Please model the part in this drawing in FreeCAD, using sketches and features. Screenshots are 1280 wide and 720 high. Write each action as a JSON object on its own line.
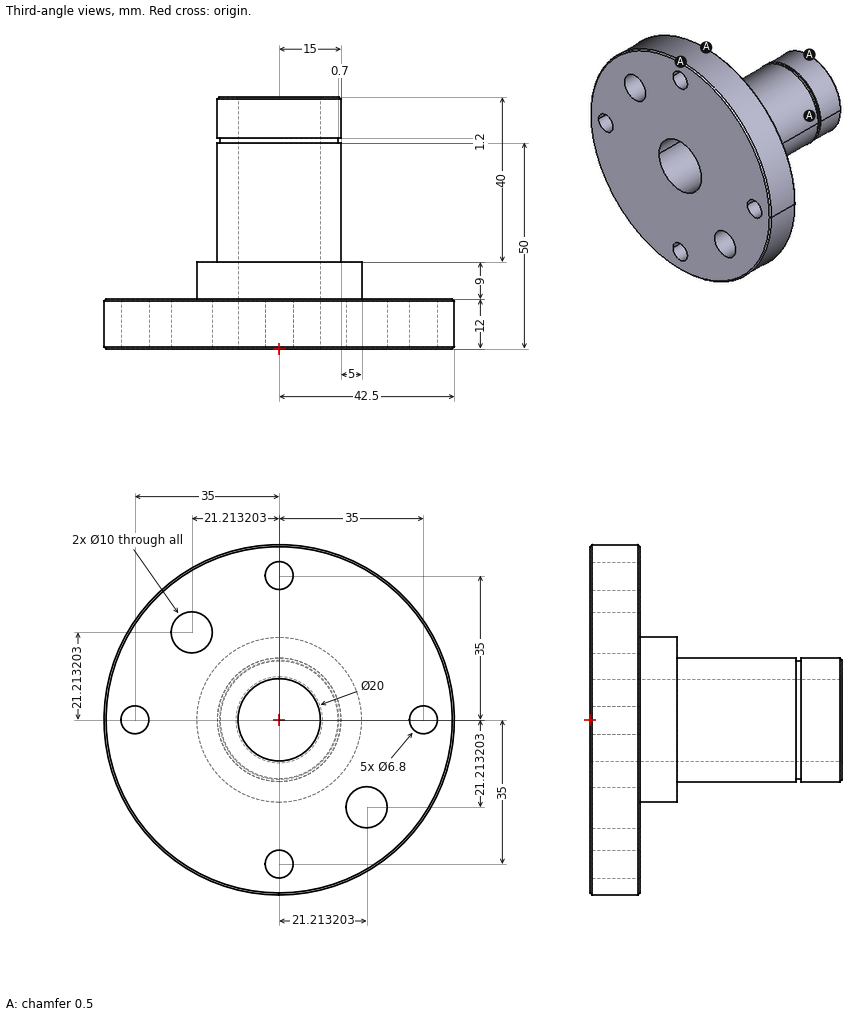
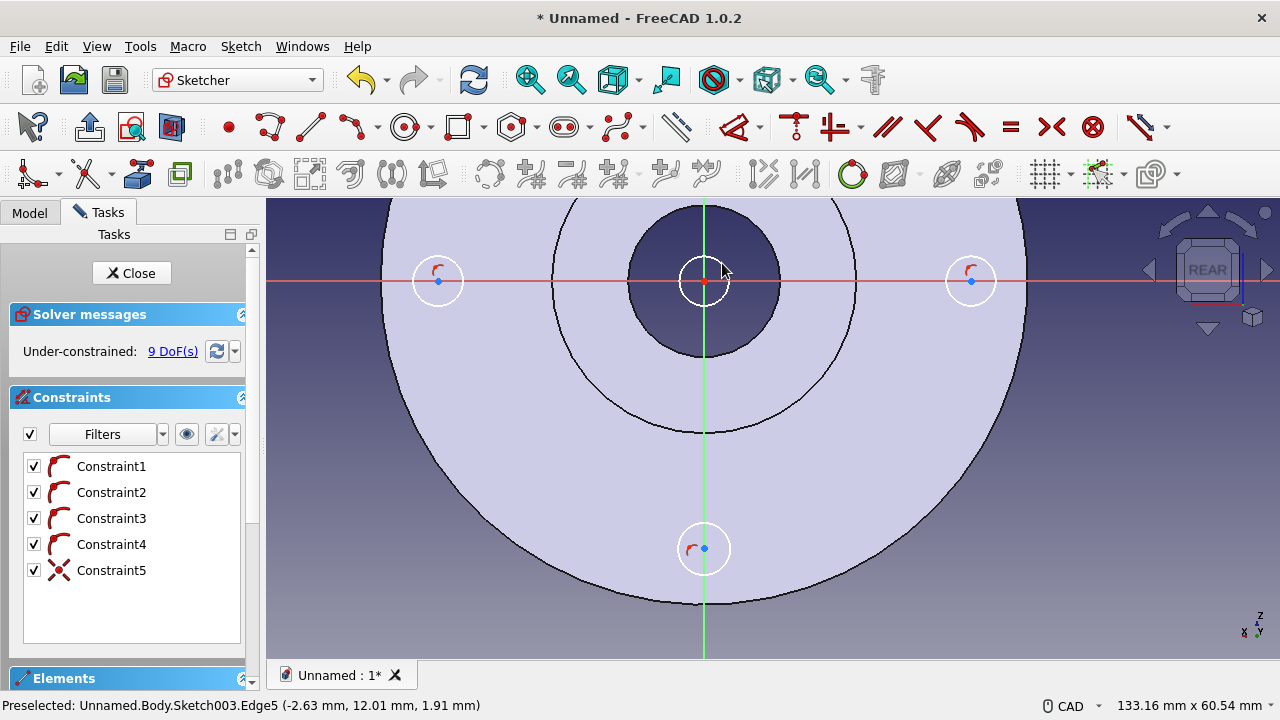
{"action": "left_click", "coordinate": [456, 263]}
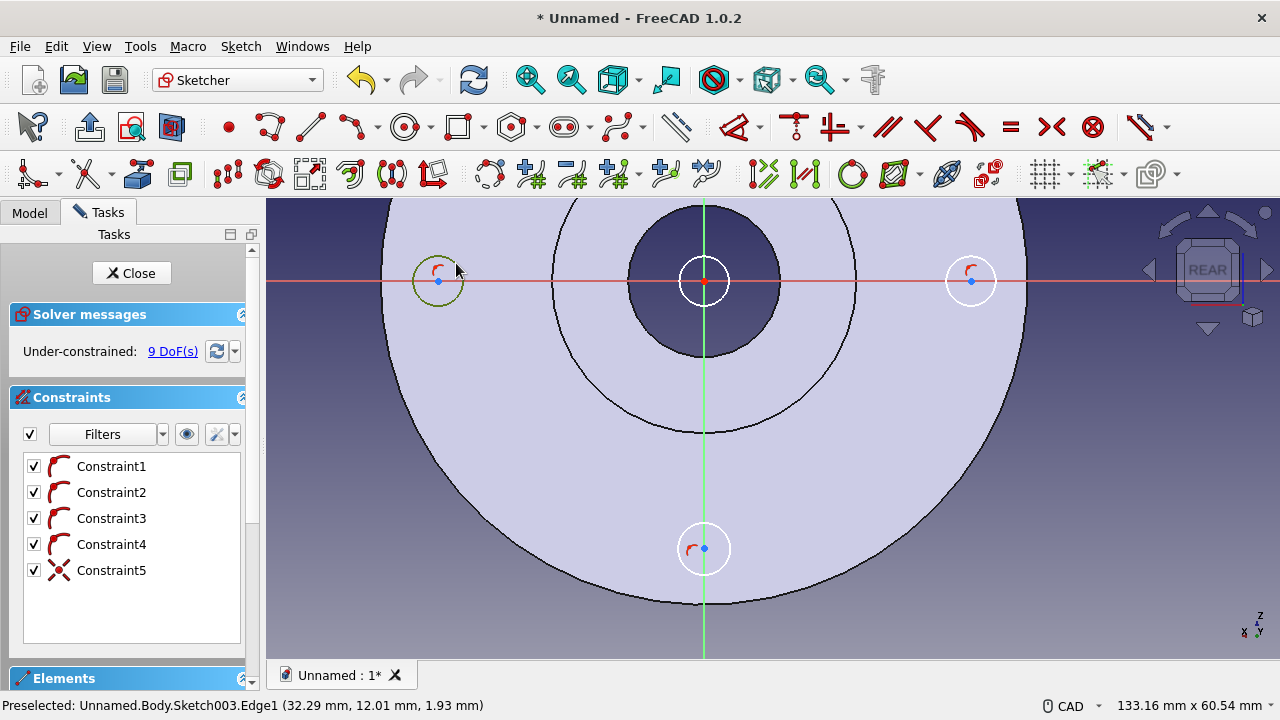
{"action": "scroll", "coordinate": [705, 549], "scroll_direction": "down", "scroll_amount": 4}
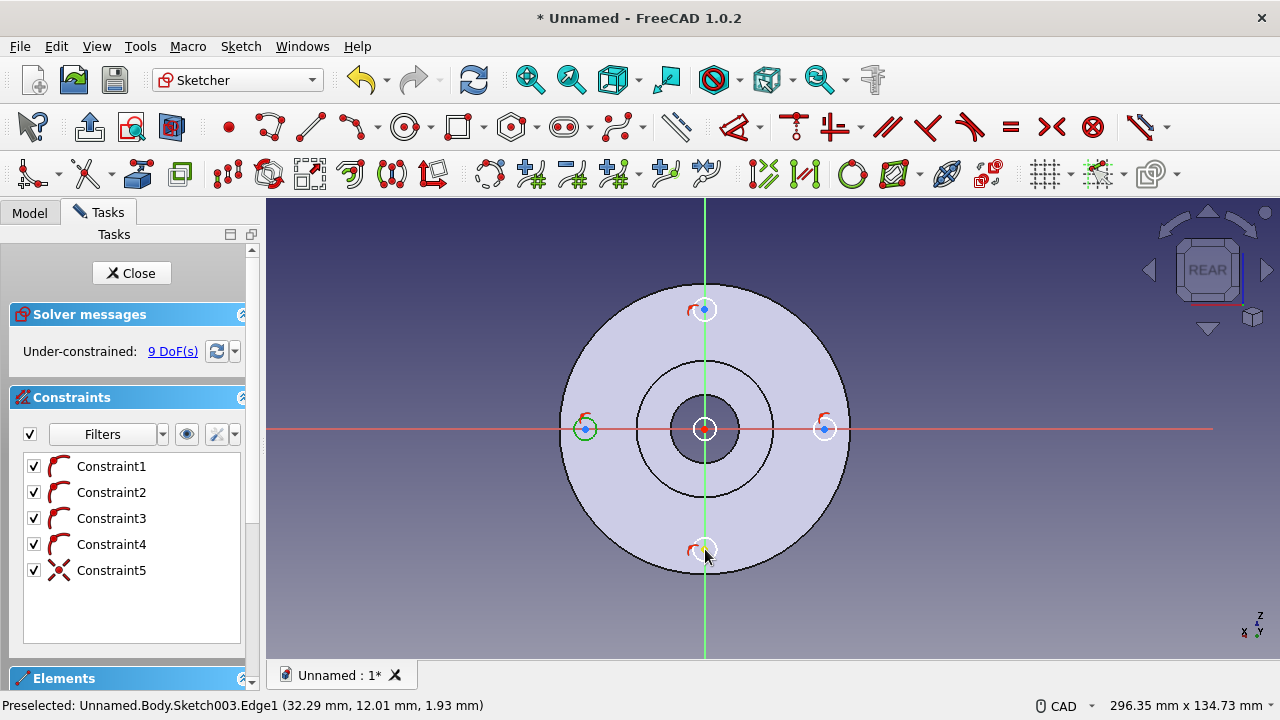
{"action": "scroll", "coordinate": [713, 302], "scroll_direction": "up", "scroll_amount": 3}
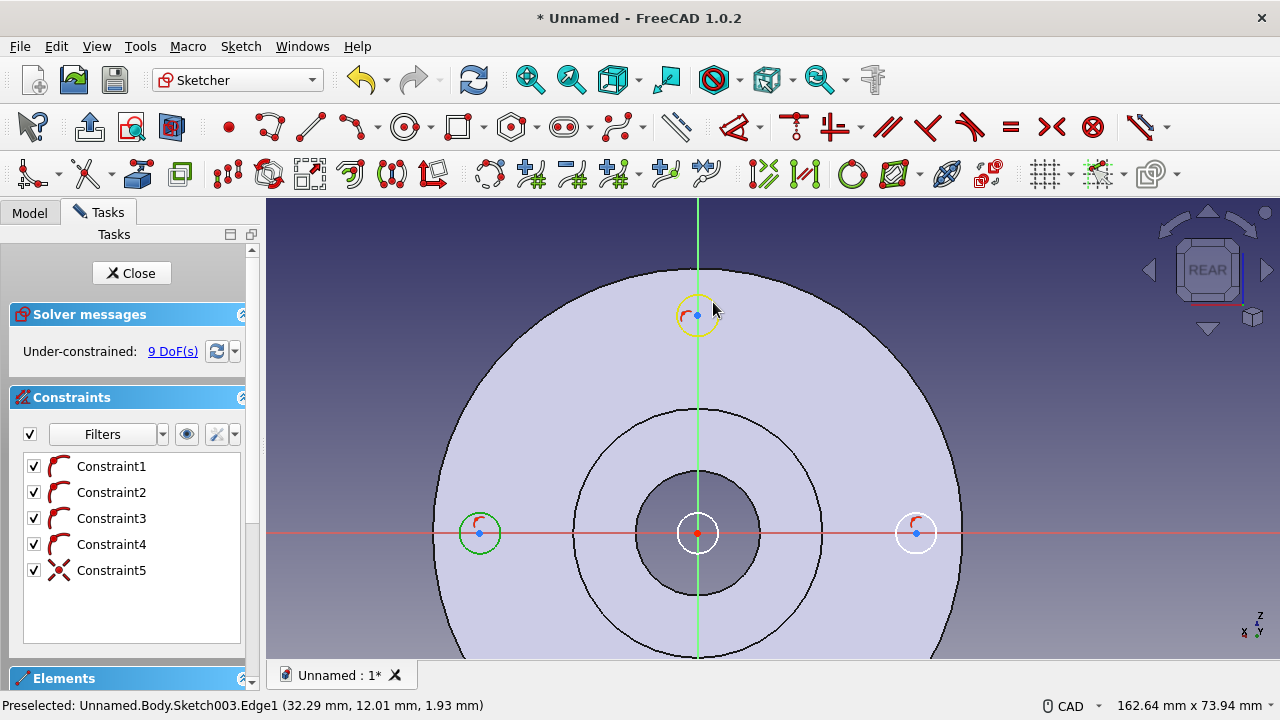
{"action": "left_click", "coordinate": [712, 301]}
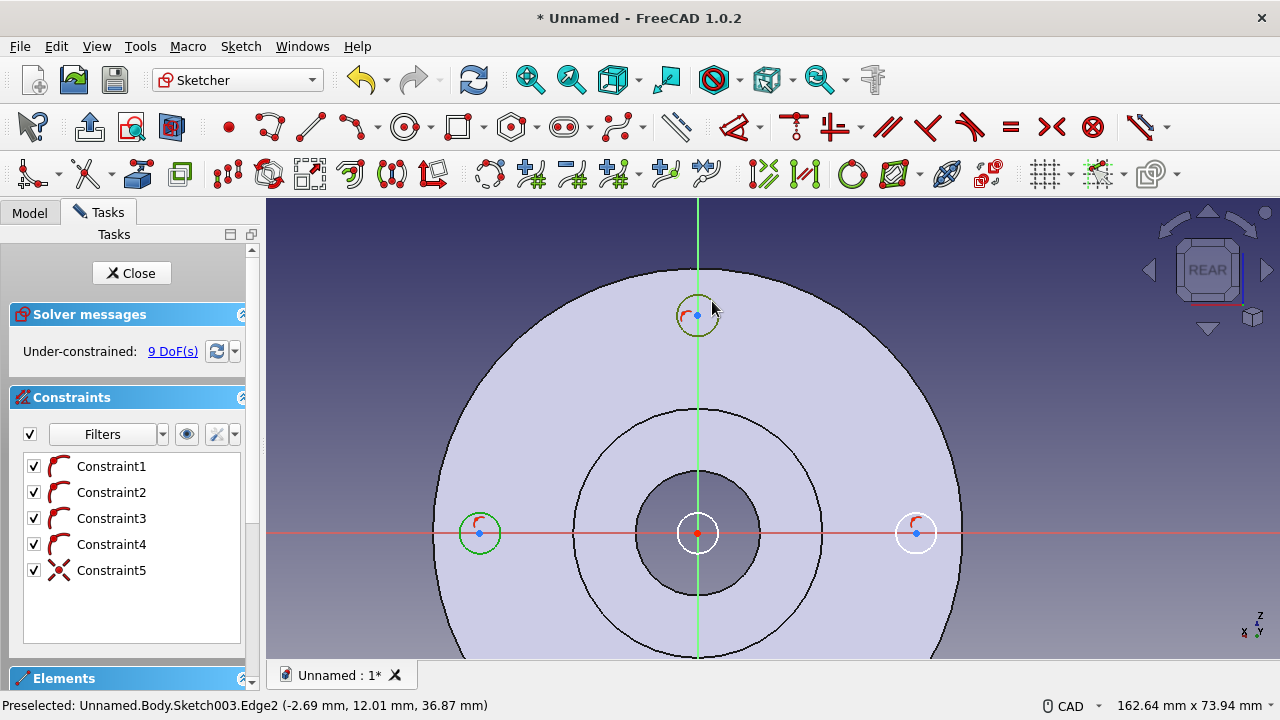
{"action": "left_click", "coordinate": [931, 519]}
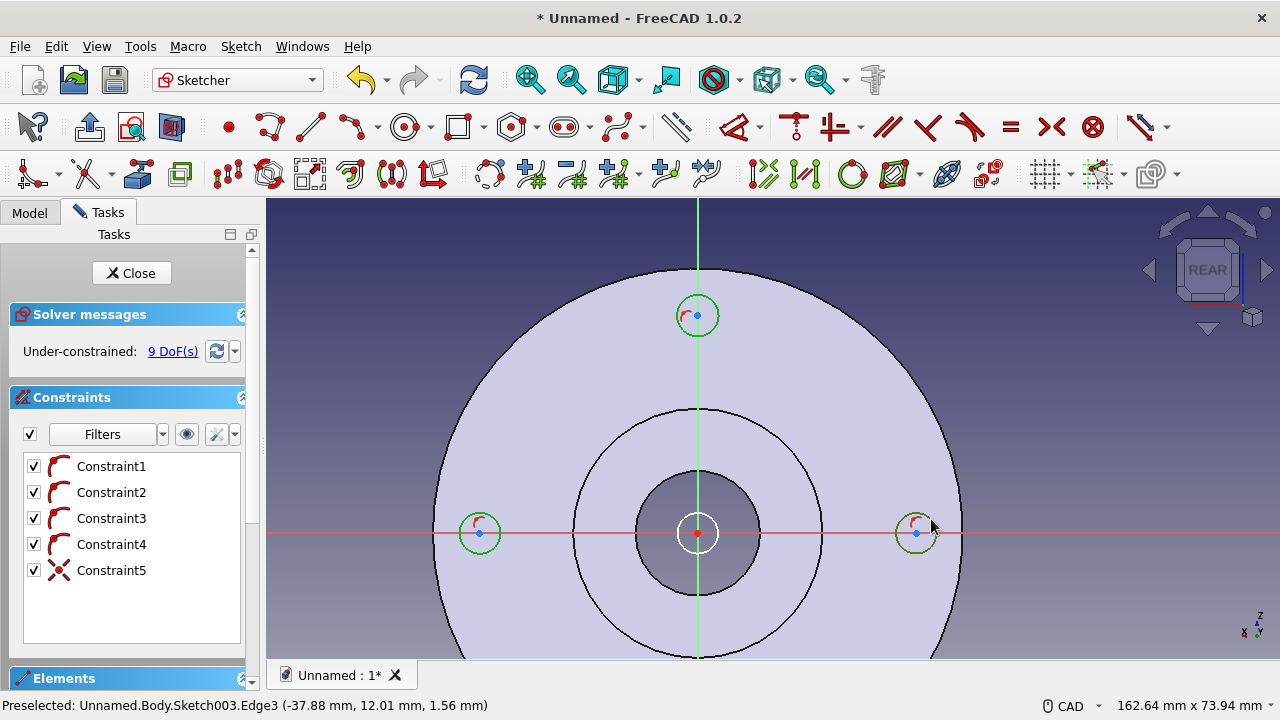
{"action": "scroll", "coordinate": [713, 301], "scroll_direction": "down", "scroll_amount": 3}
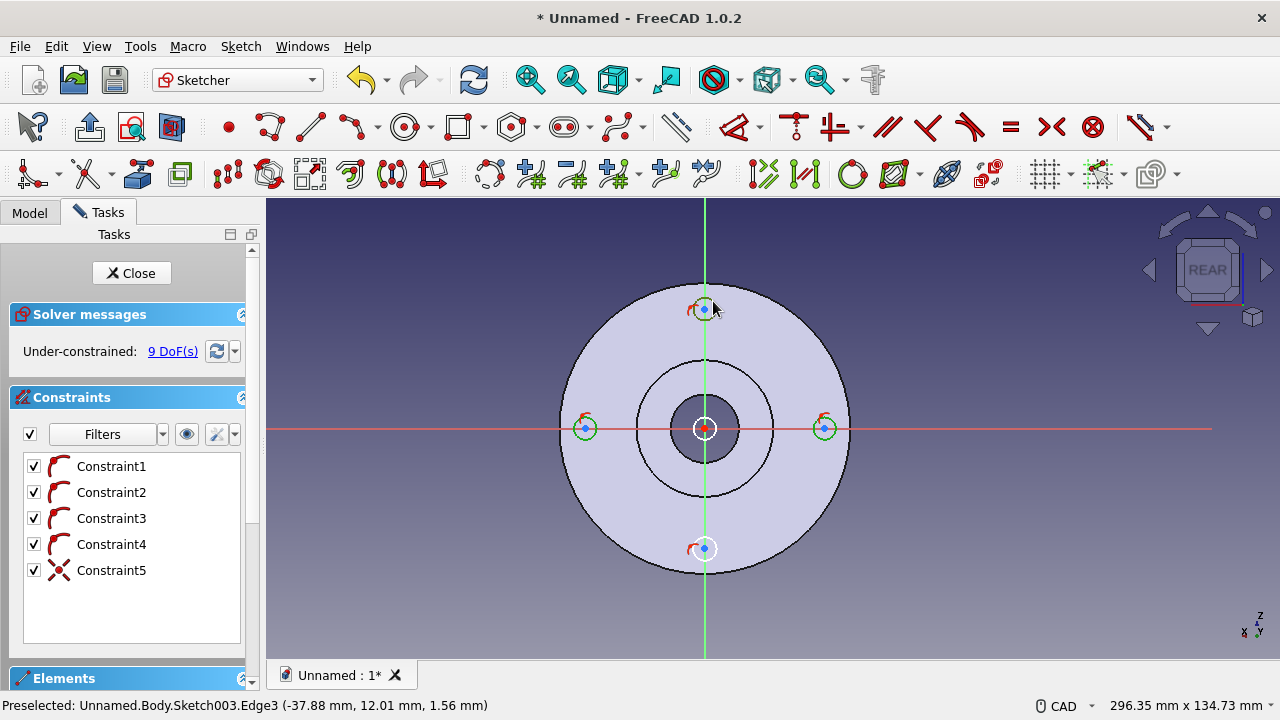
{"action": "scroll", "coordinate": [713, 541], "scroll_direction": "up", "scroll_amount": 3}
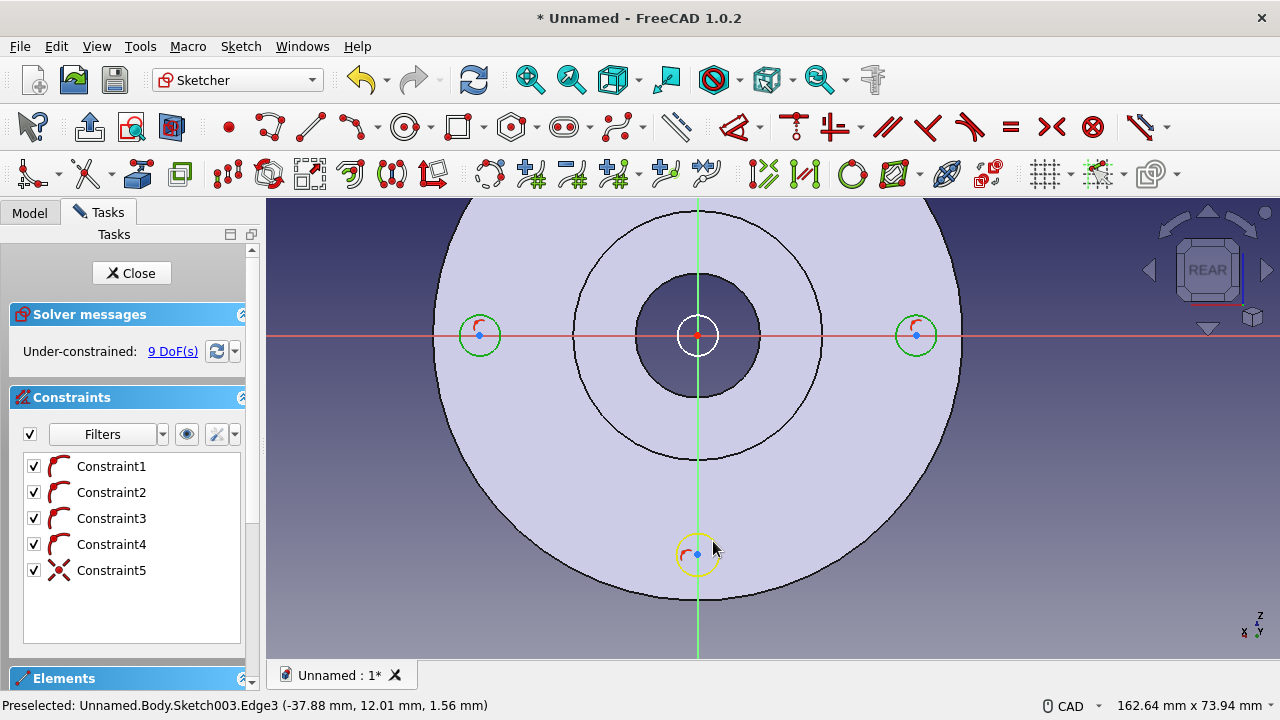
{"action": "left_click", "coordinate": [713, 540]}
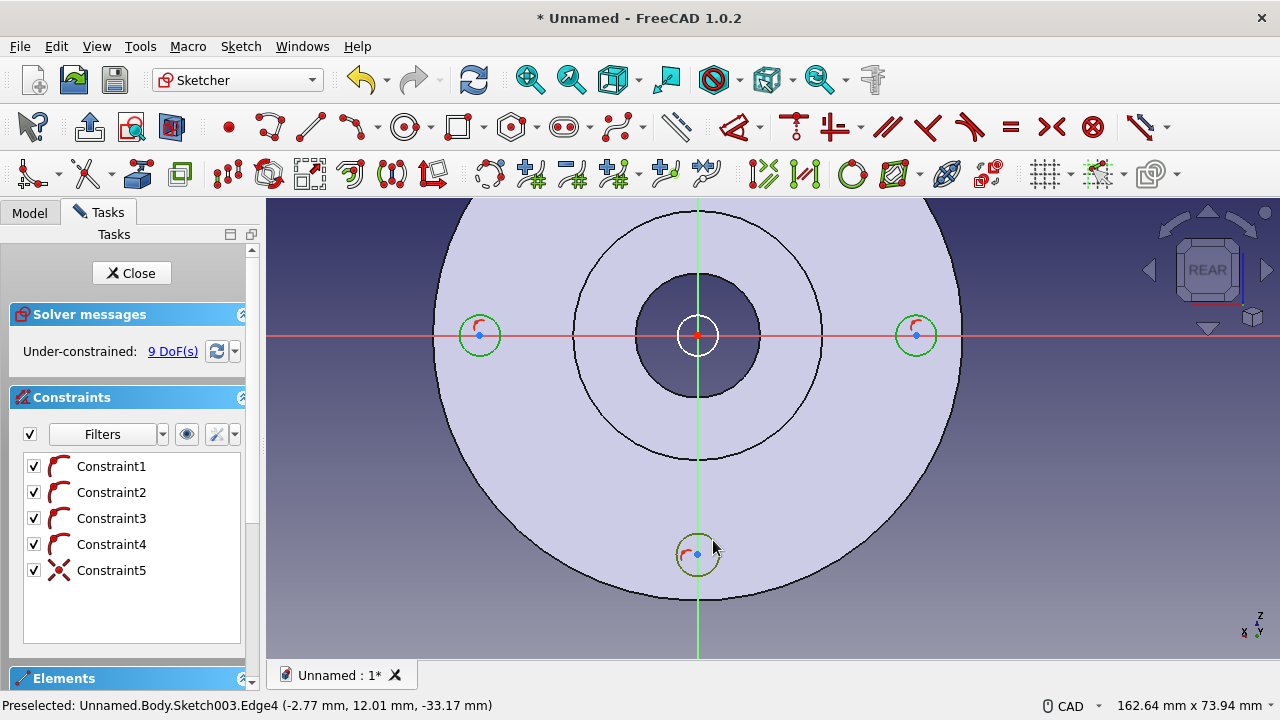
{"action": "left_click", "coordinate": [712, 321]}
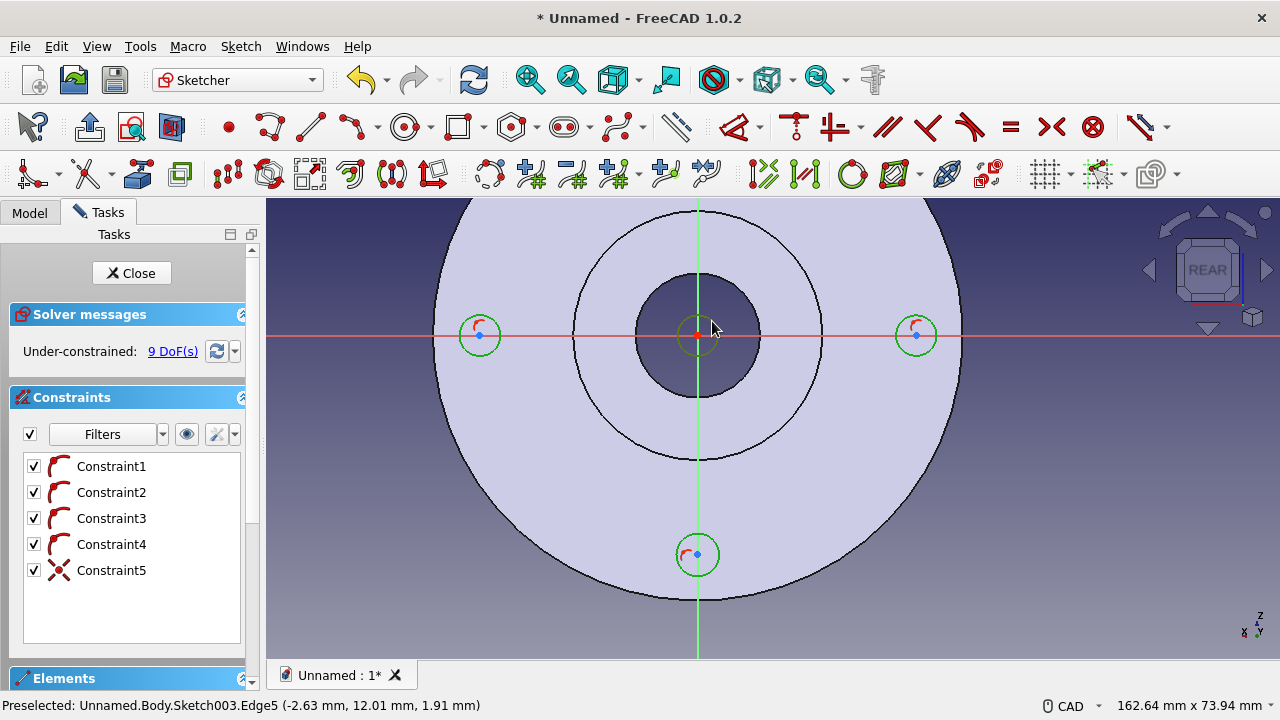
{"action": "left_click", "coordinate": [1011, 128]}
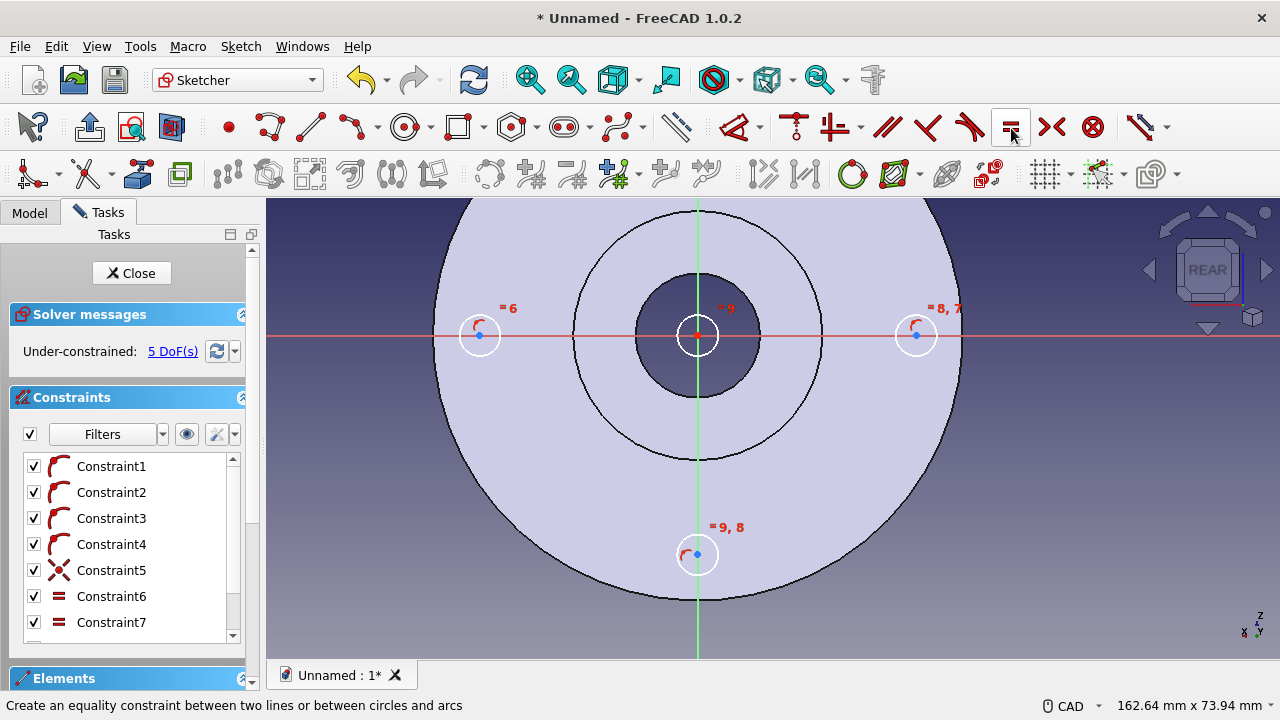
{"action": "left_click", "coordinate": [734, 128]}